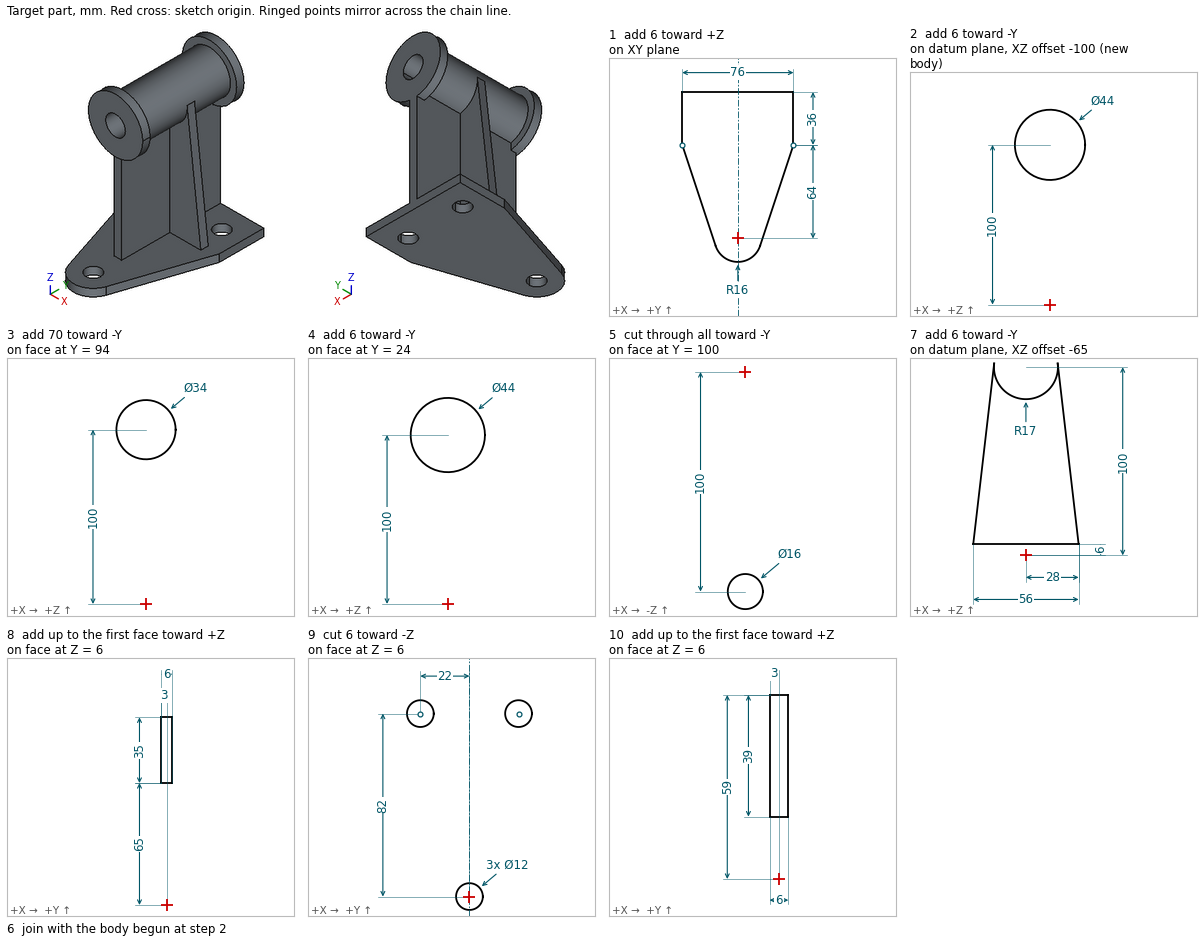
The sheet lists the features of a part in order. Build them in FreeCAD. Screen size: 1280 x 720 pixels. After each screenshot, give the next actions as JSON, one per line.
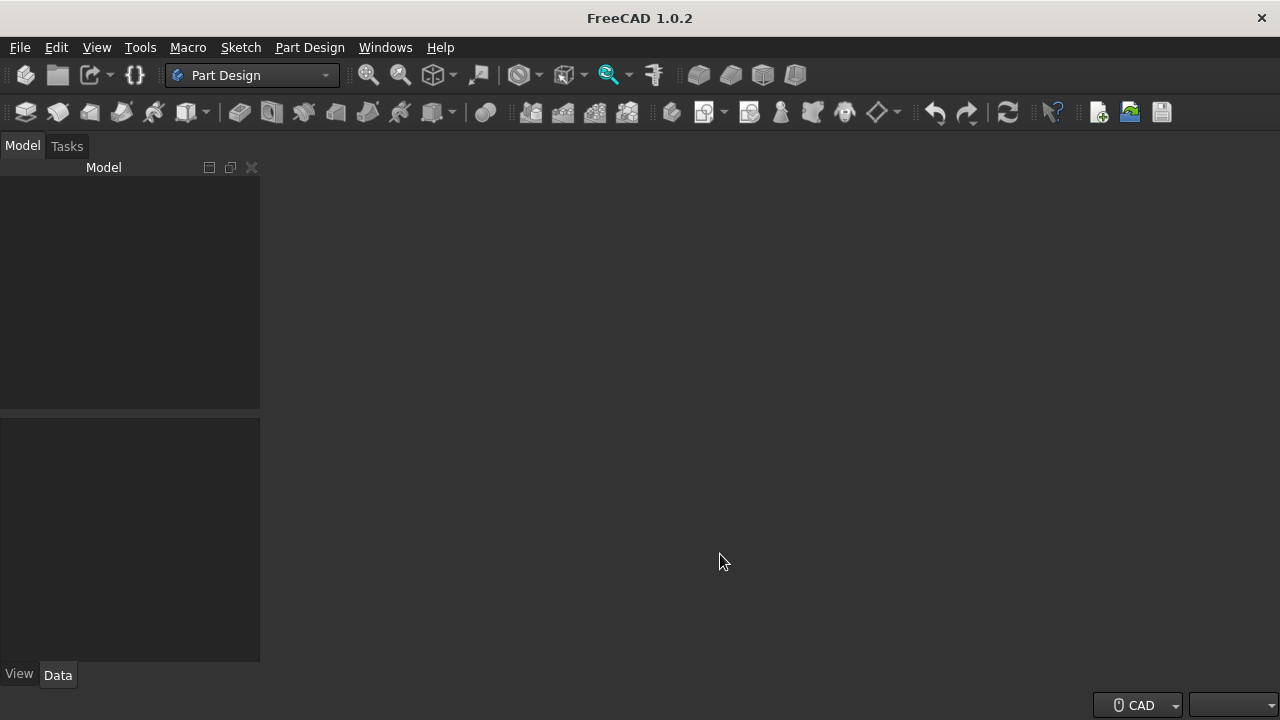
{"action": "key", "text": "ctrl+n"}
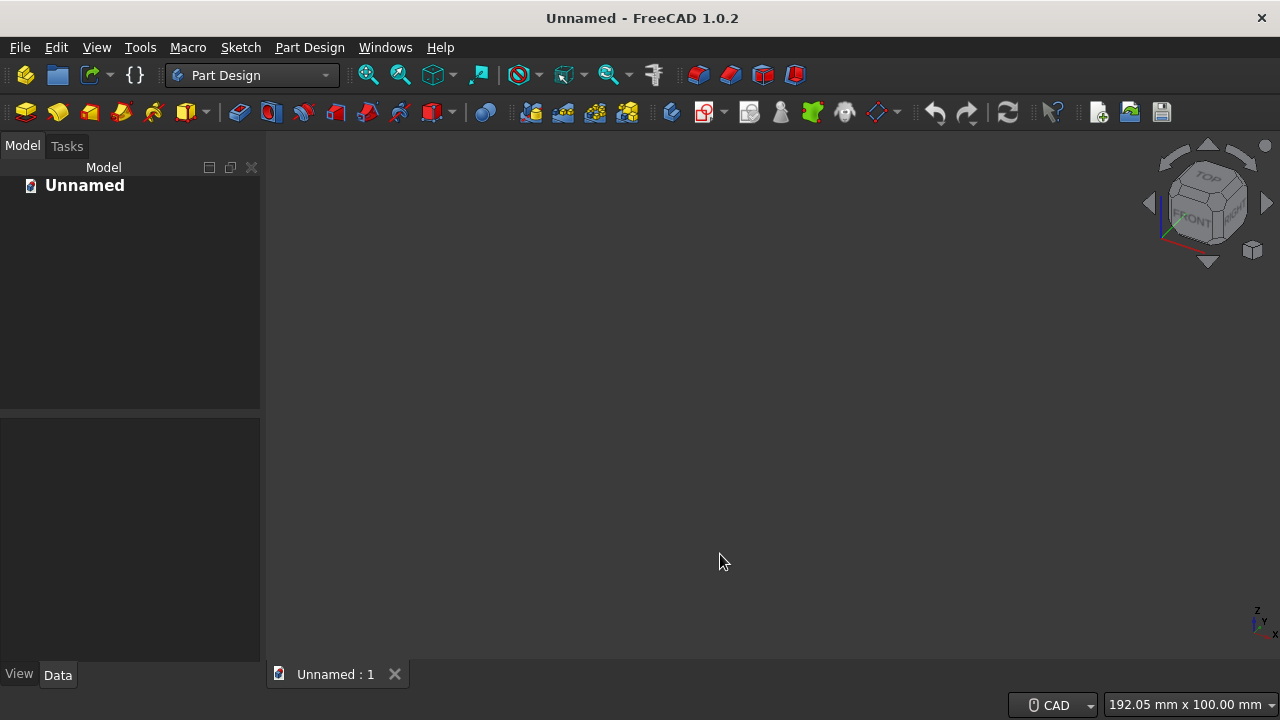
{"action": "left_click", "coordinate": [704, 112]}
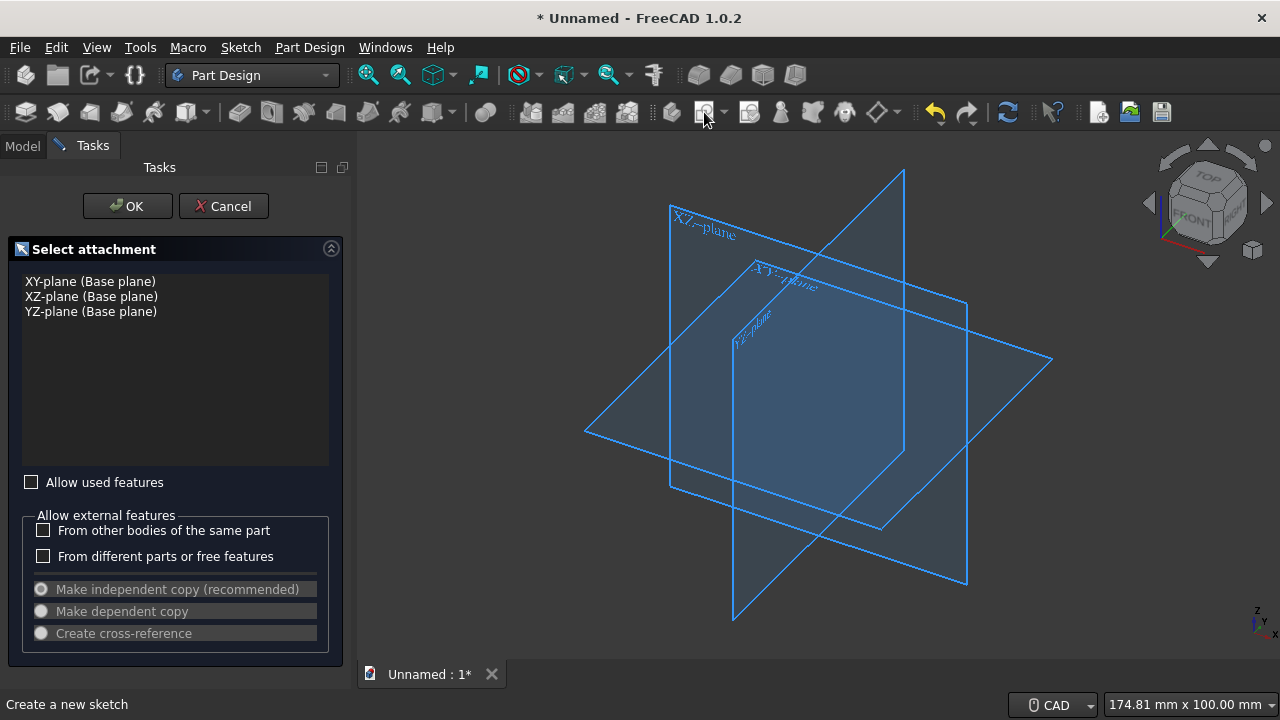
{"action": "left_click", "coordinate": [82, 282]}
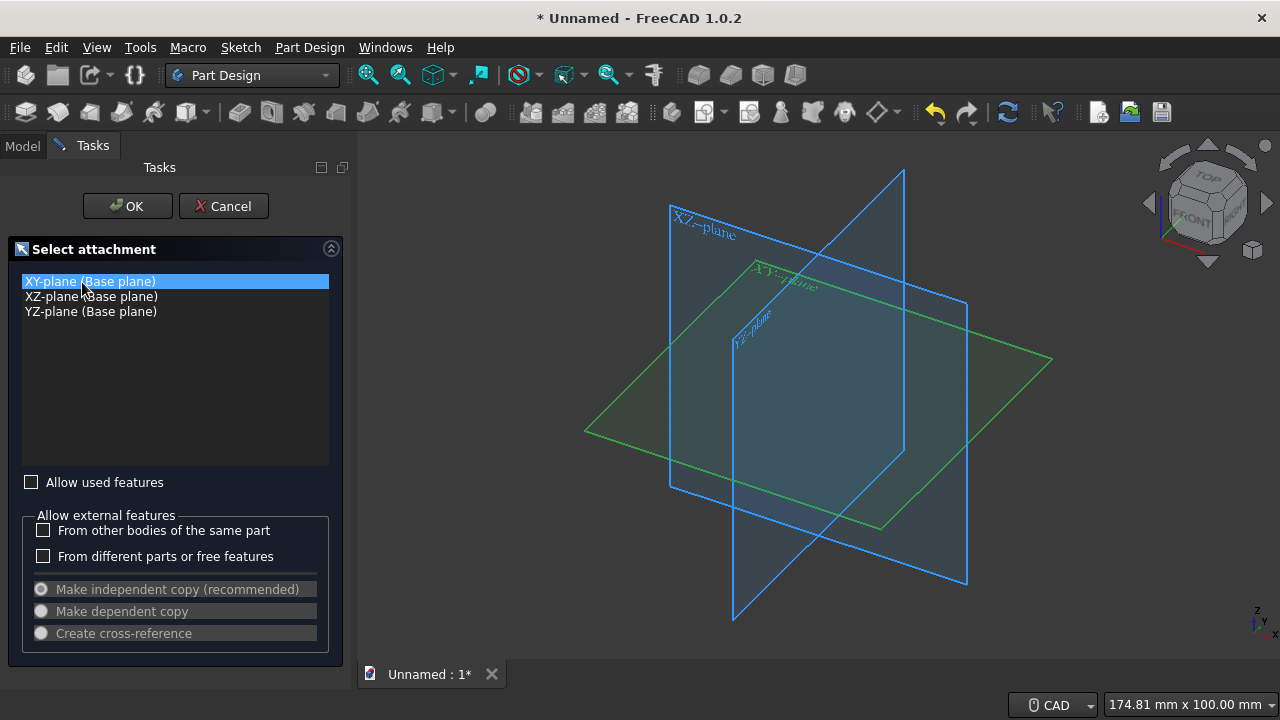
{"action": "left_click", "coordinate": [128, 206]}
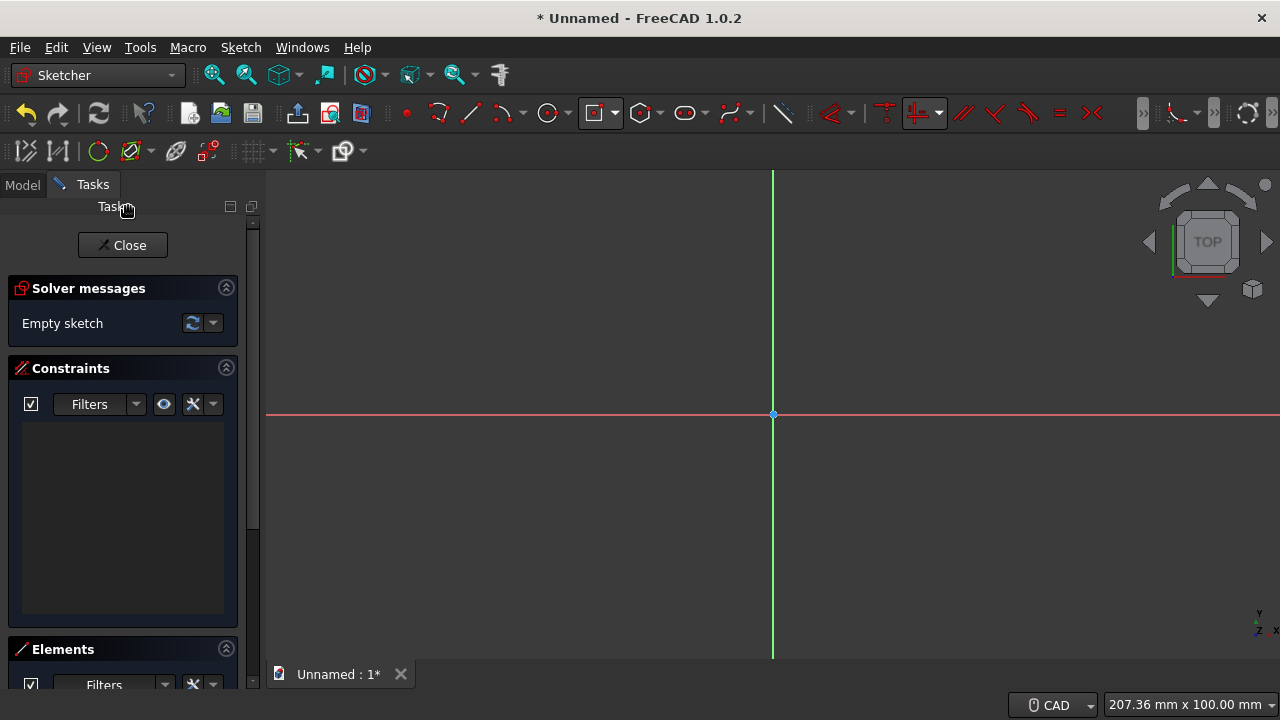
{"action": "scroll", "coordinate": [621, 631], "scroll_direction": "down", "scroll_amount": 3}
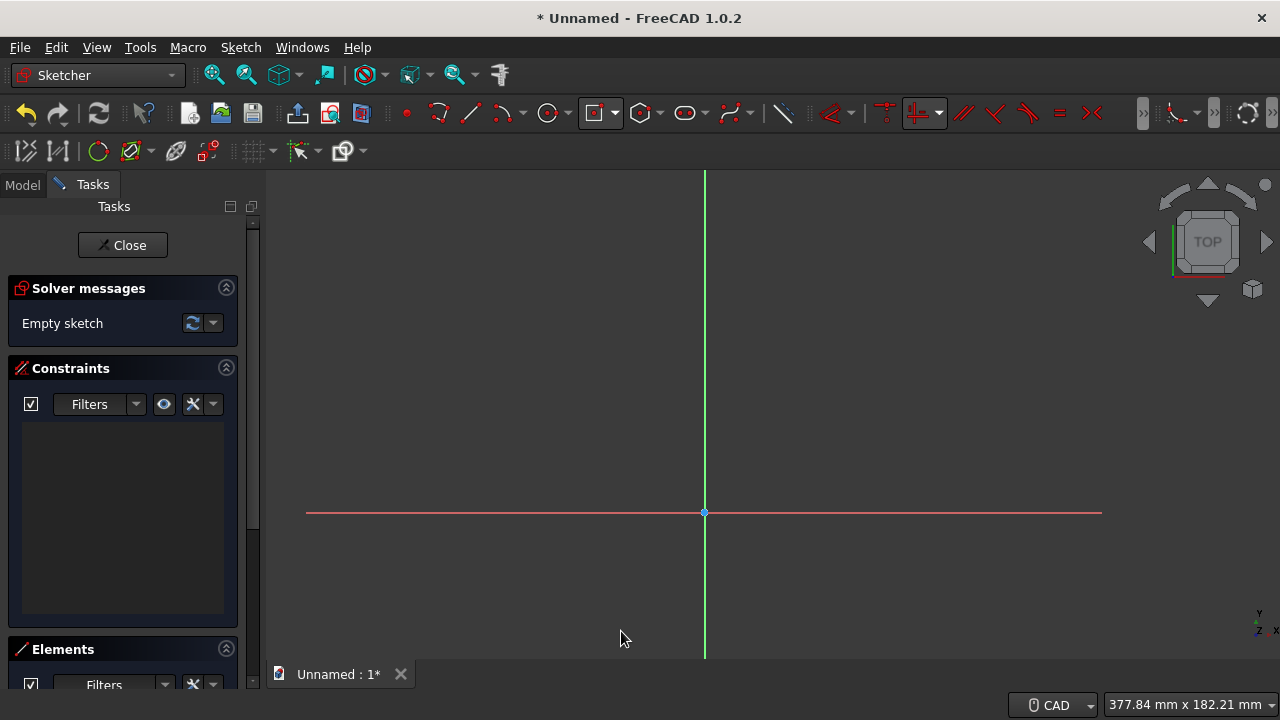
{"action": "key", "text": "g m"}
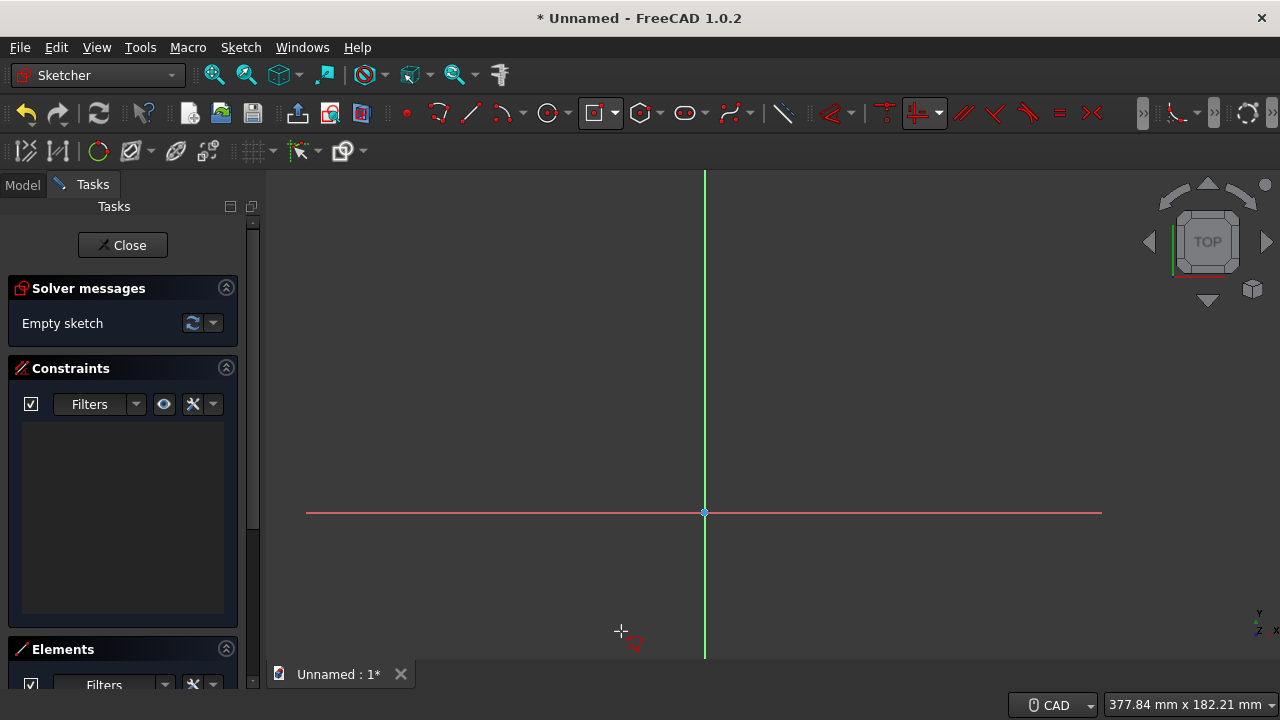
{"action": "left_click", "coordinate": [745, 526]}
{"action": "left_click", "coordinate": [807, 341]}
{"action": "left_click", "coordinate": [807, 244]}
{"action": "left_click", "coordinate": [603, 244]}
{"action": "left_click", "coordinate": [603, 341]}
{"action": "left_click", "coordinate": [664, 526]}
{"action": "right_click", "coordinate": [664, 526]}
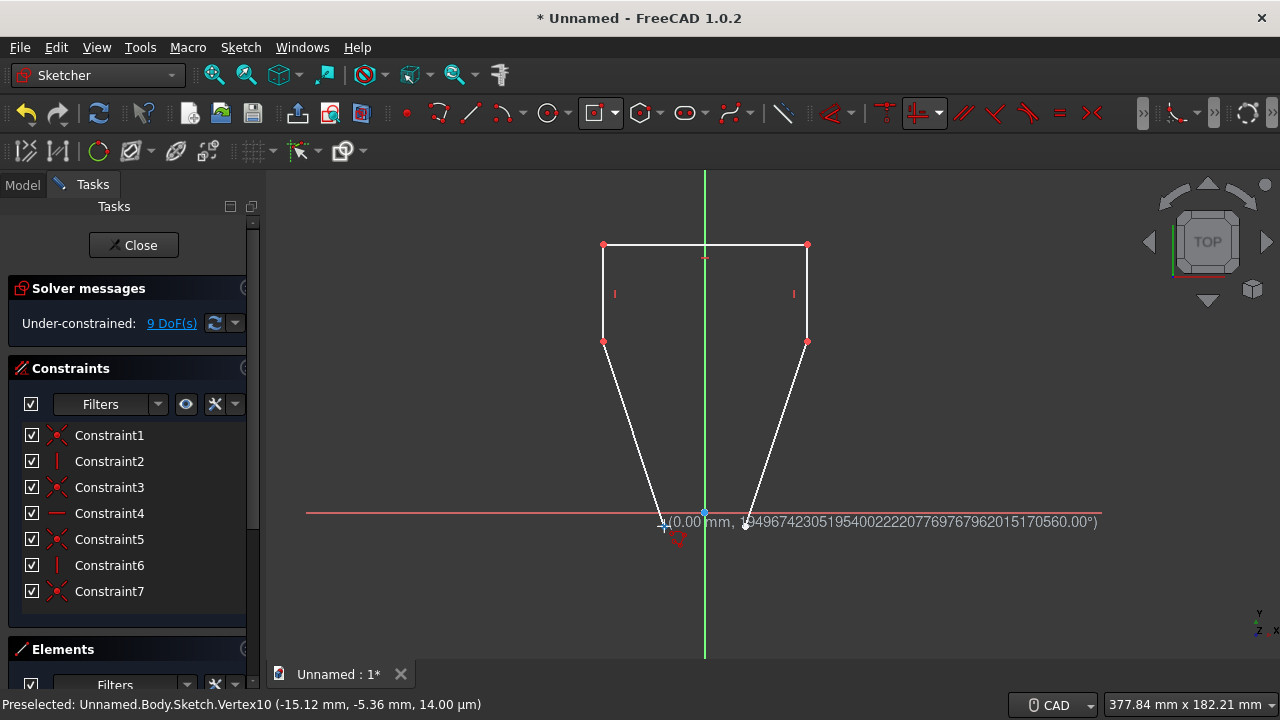
{"action": "key", "text": "g 3 a"}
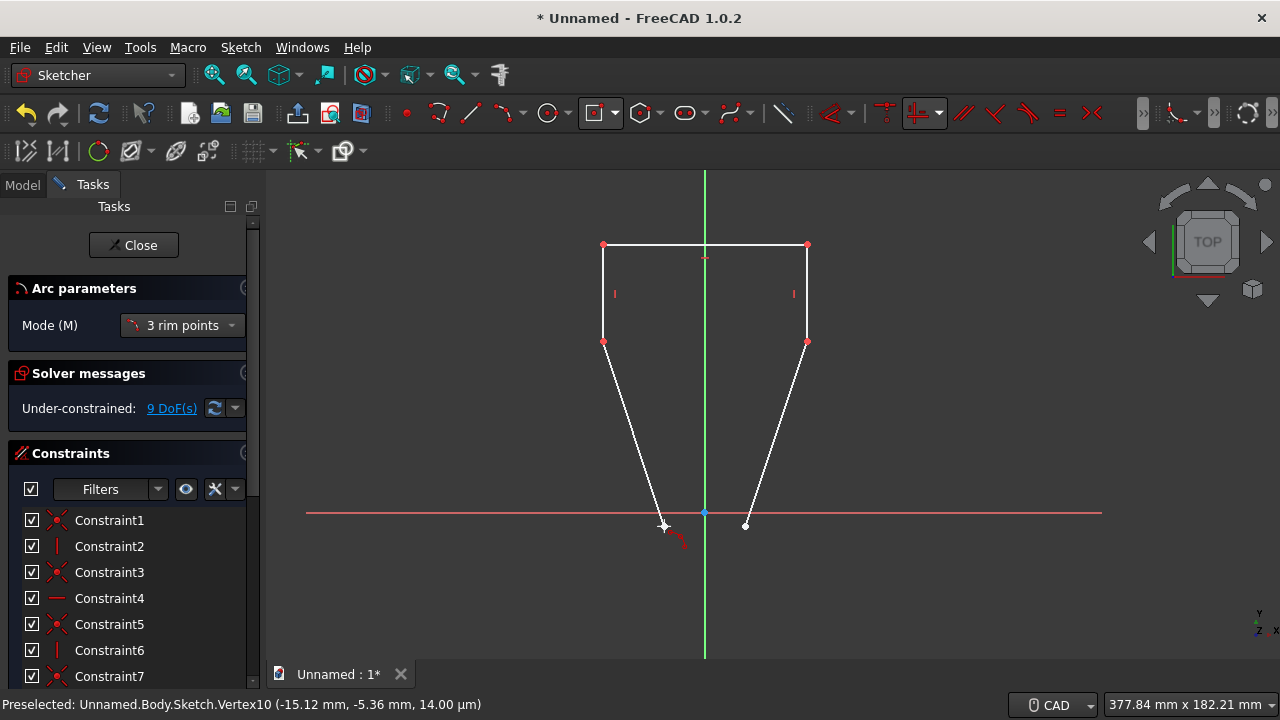
{"action": "left_click", "coordinate": [664, 527]}
{"action": "left_click", "coordinate": [745, 527]}
{"action": "left_click", "coordinate": [684, 550]}
{"action": "key", "text": "Escape"}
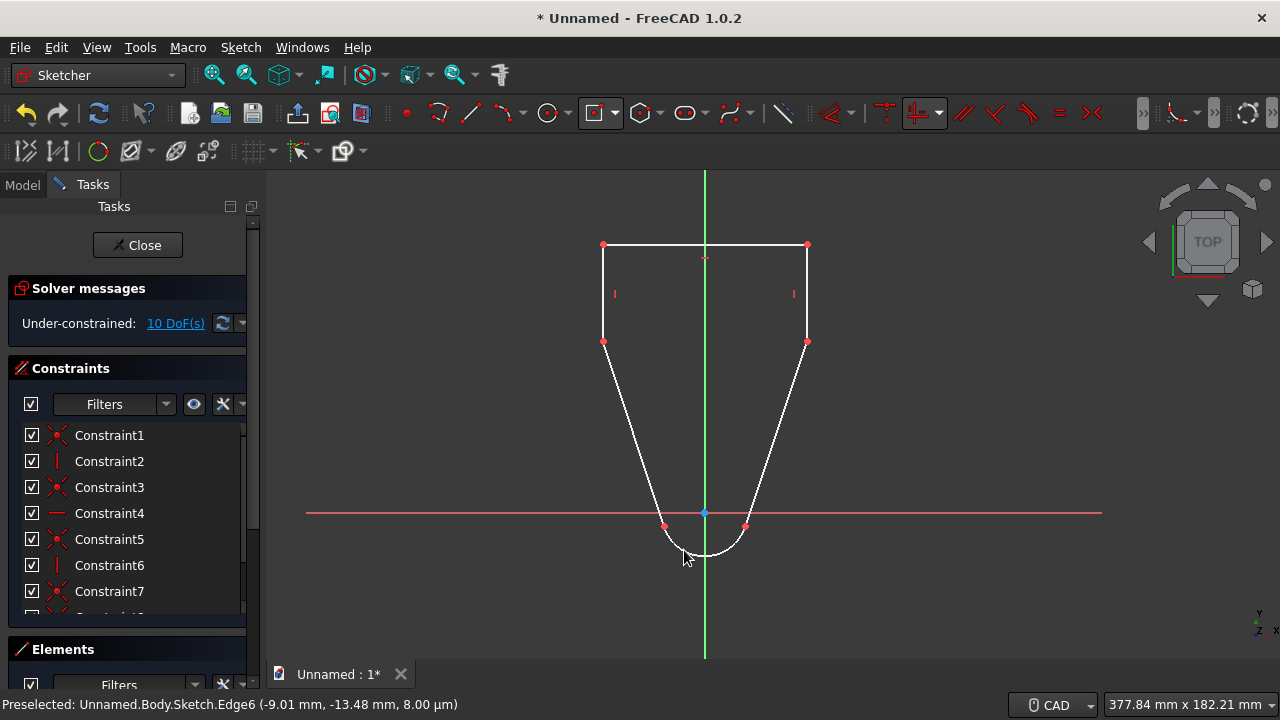
{"action": "left_click", "coordinate": [764, 471]}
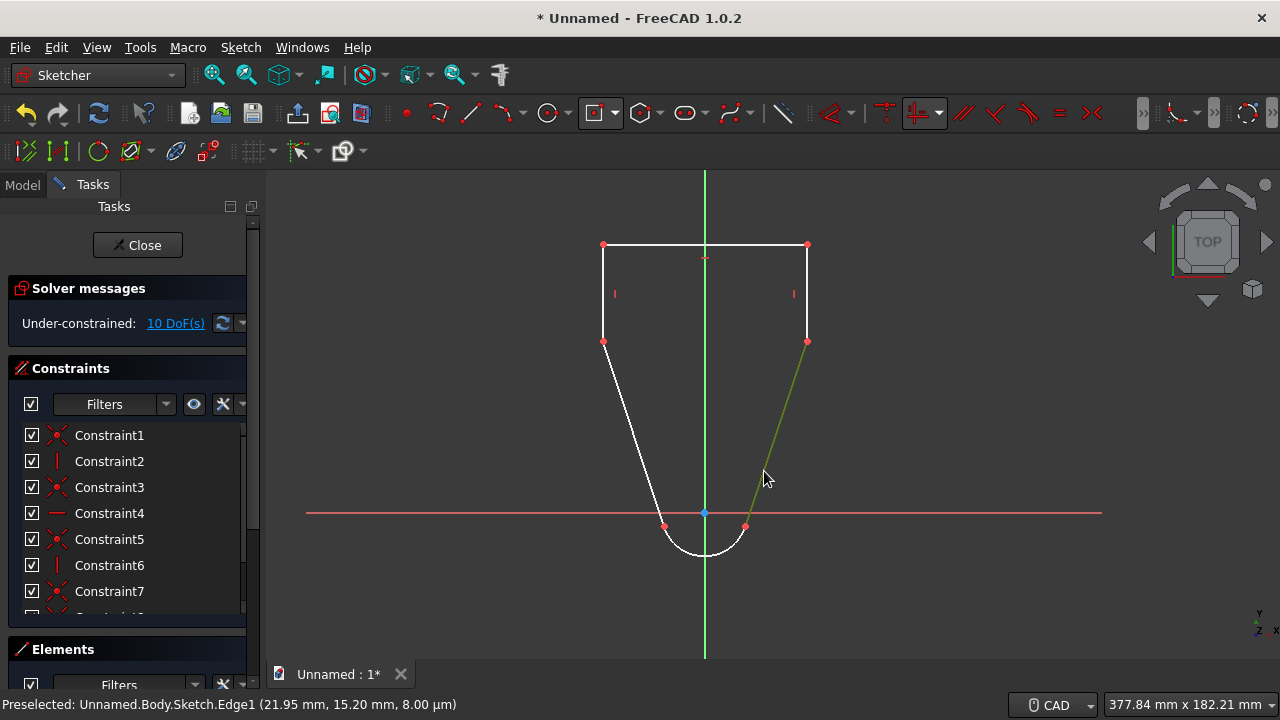
{"action": "left_click", "coordinate": [684, 551]}